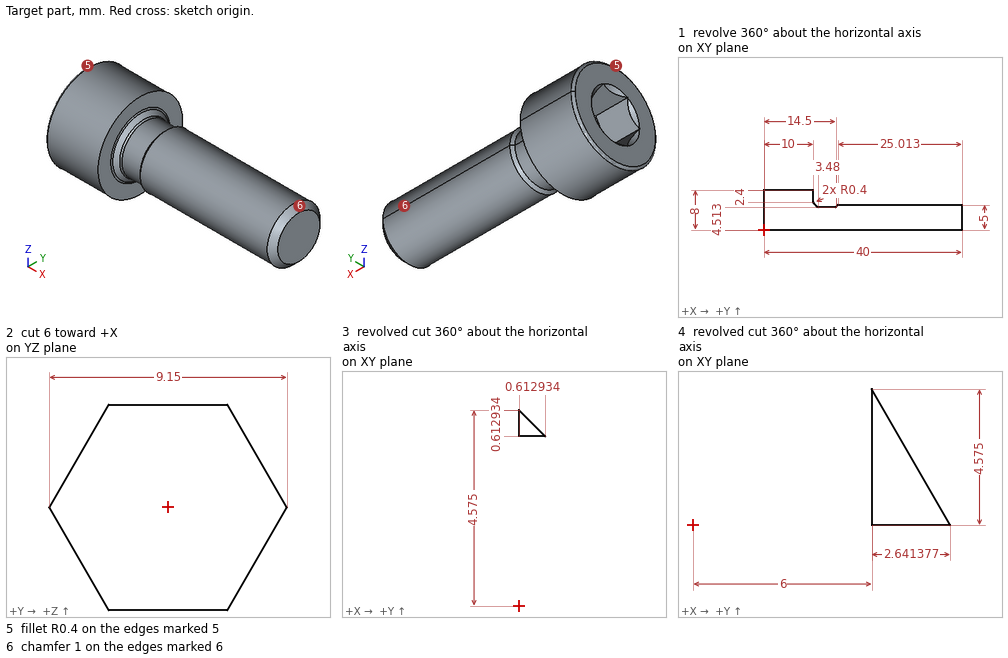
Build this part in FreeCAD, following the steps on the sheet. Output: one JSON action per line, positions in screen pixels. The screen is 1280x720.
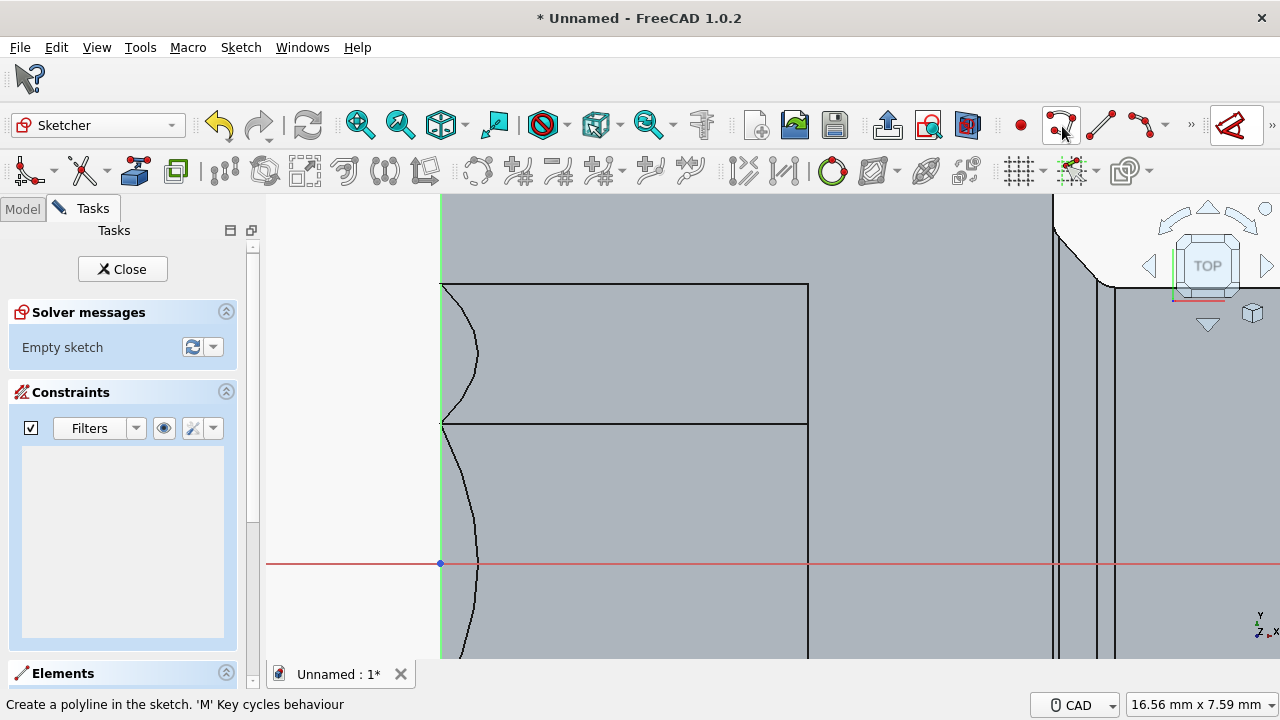
{"action": "left_click", "coordinate": [808, 564]}
{"action": "left_click", "coordinate": [970, 555]}
{"action": "left_click", "coordinate": [808, 284]}
{"action": "left_click", "coordinate": [808, 564]}
{"action": "key", "text": "Escape"}
{"action": "key", "text": "Escape"}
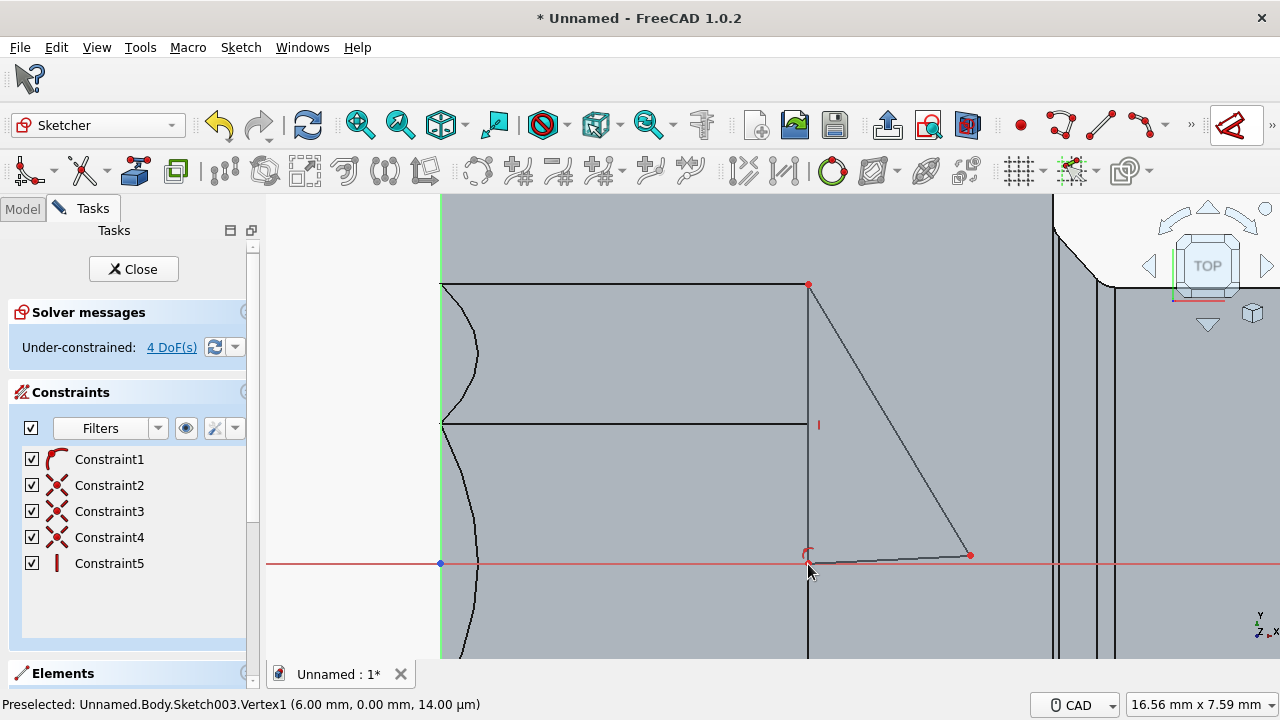
{"action": "left_click", "coordinate": [857, 561]}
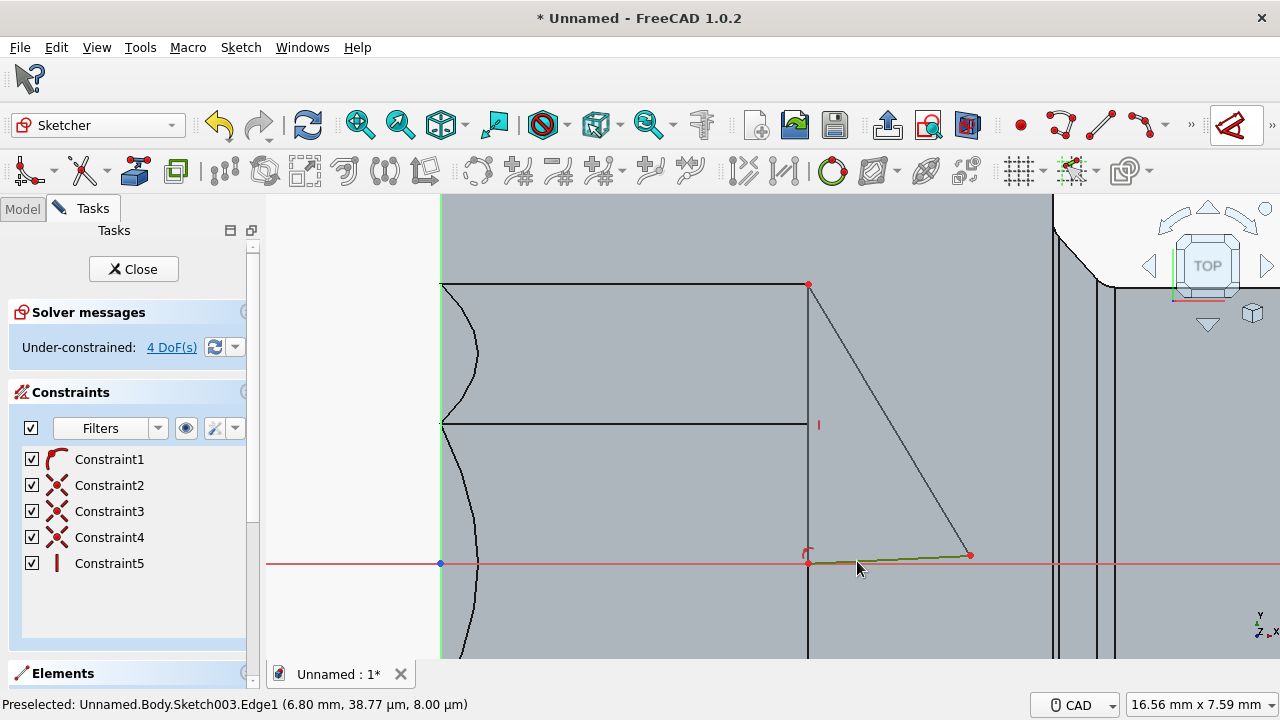
{"action": "key", "text": "h"}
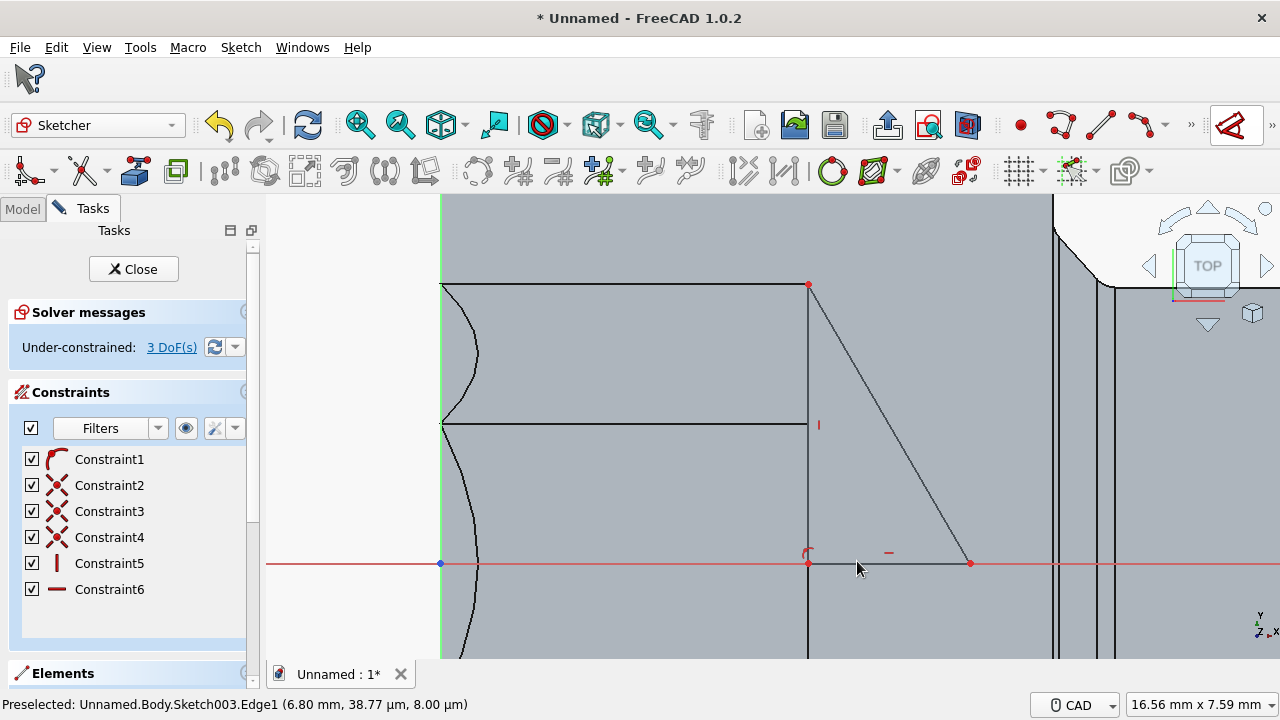
{"action": "left_click", "coordinate": [808, 564]}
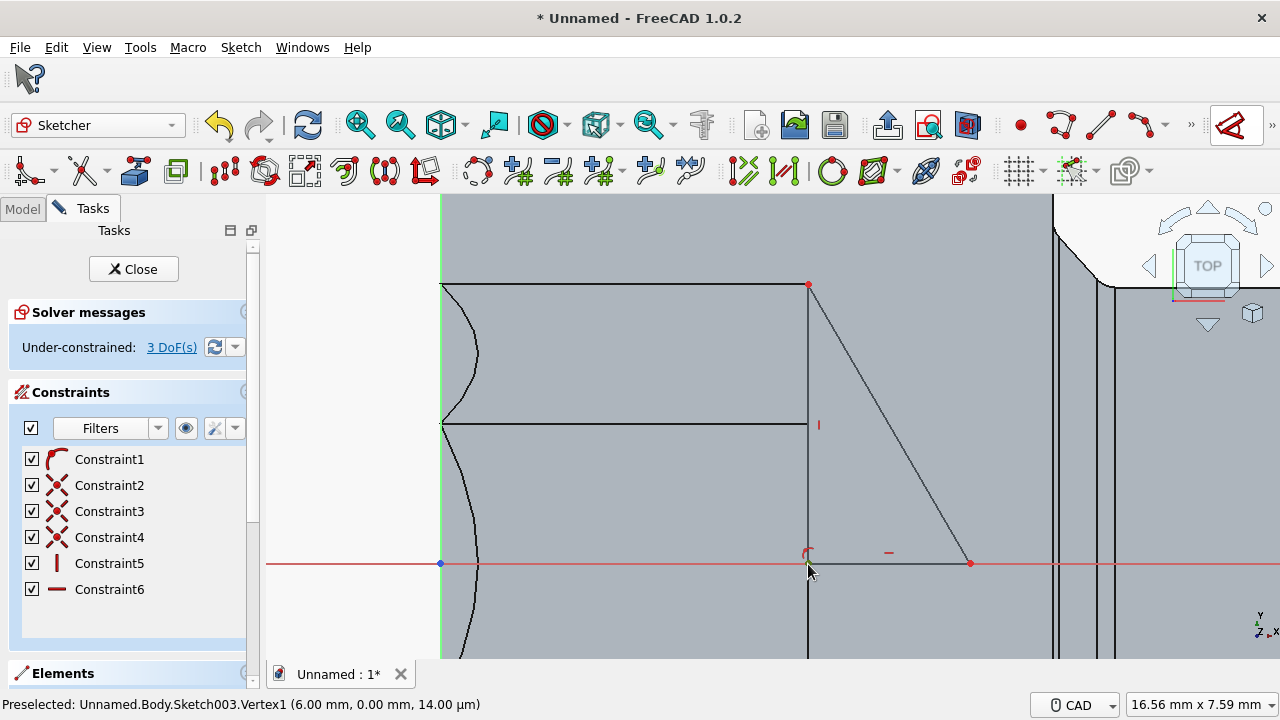
{"action": "left_click", "coordinate": [1258, 126]}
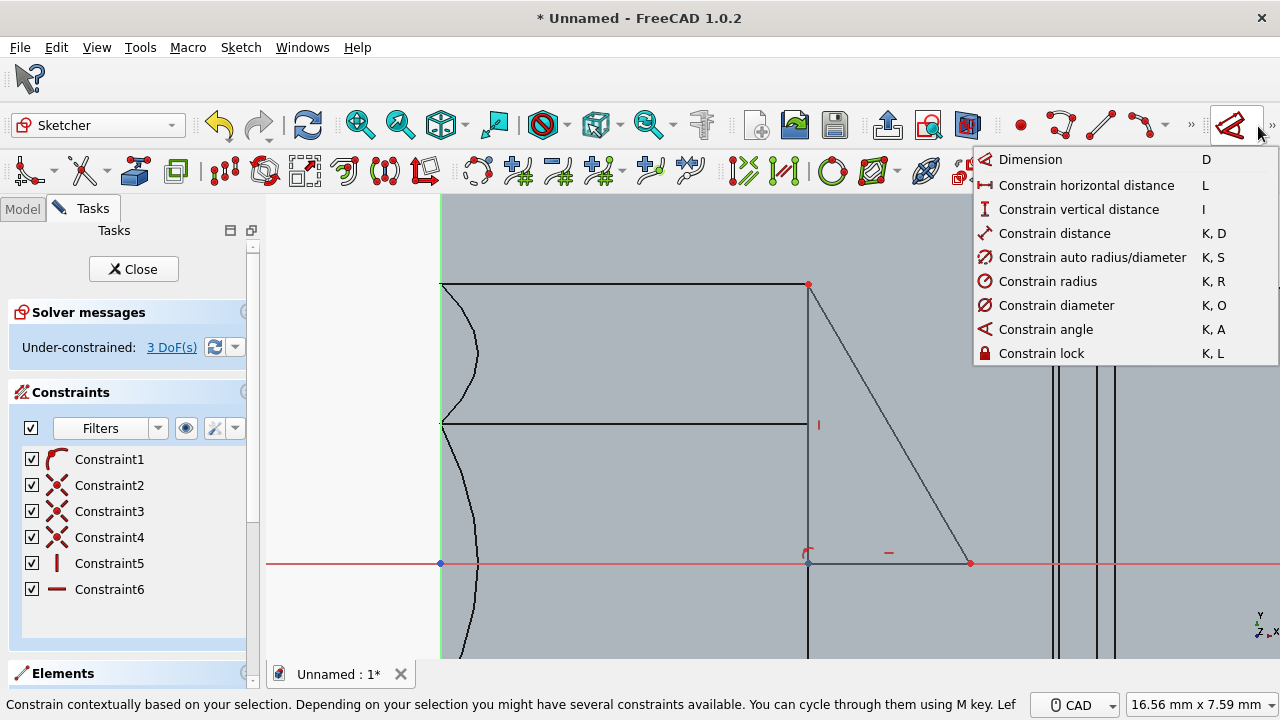
{"action": "left_click", "coordinate": [1126, 185]}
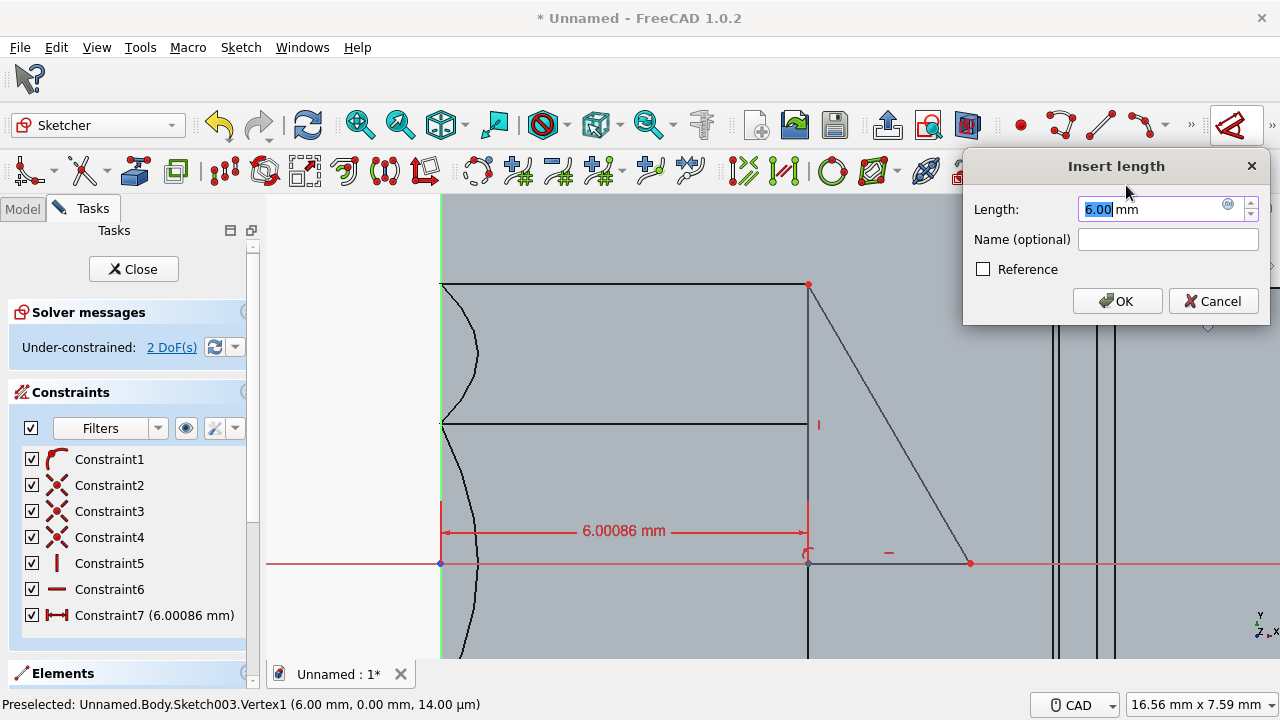
{"action": "type", "text": "6"}
{"action": "key", "text": "Return"}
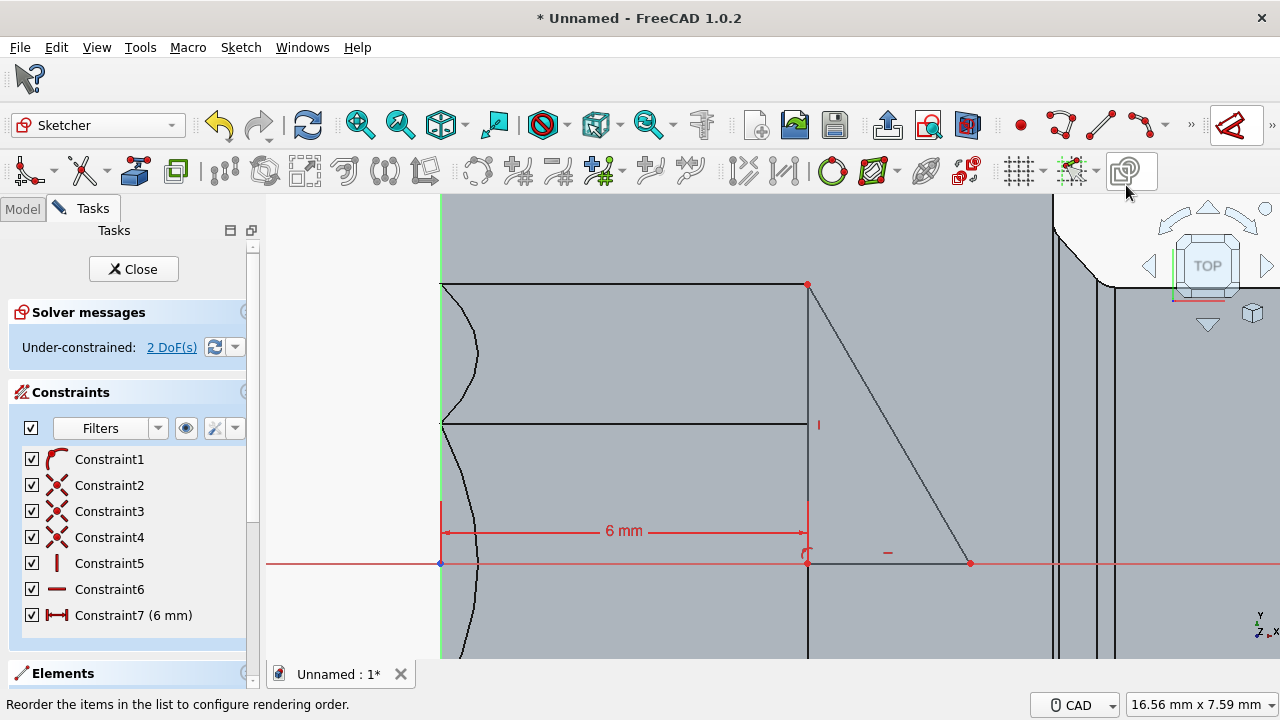
{"action": "left_click", "coordinate": [808, 369]}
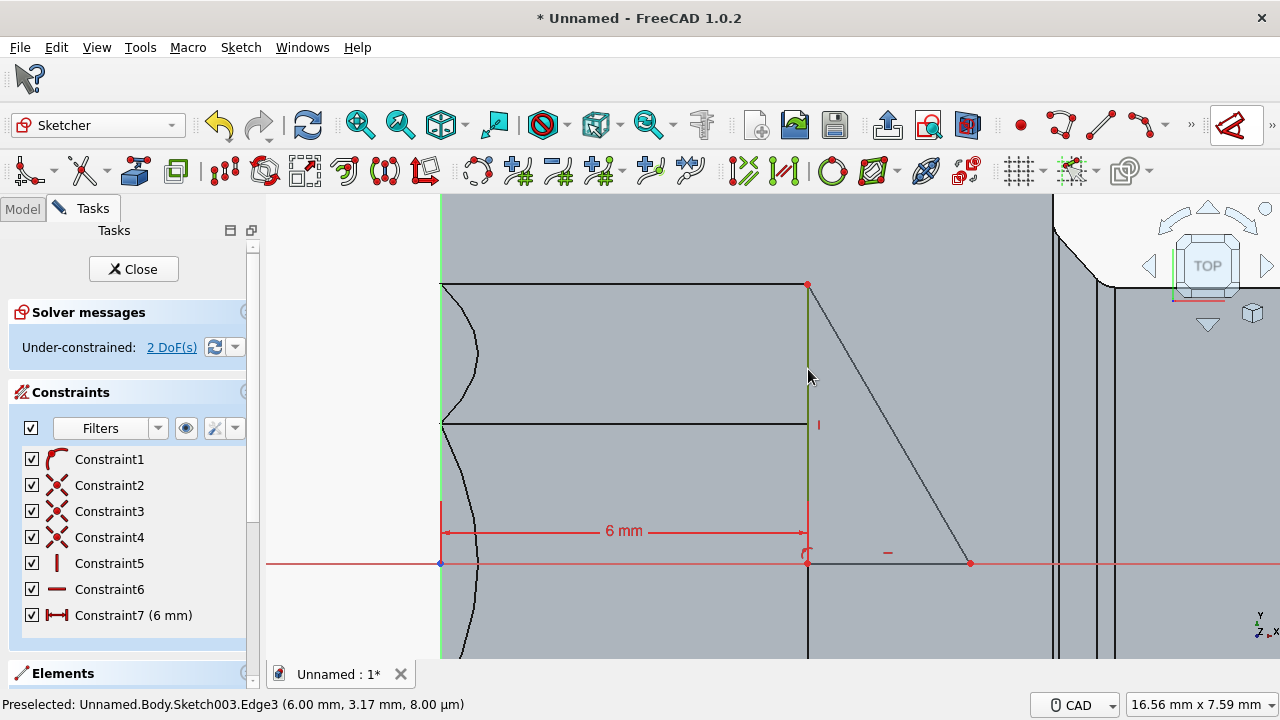
{"action": "left_click", "coordinate": [1258, 126]}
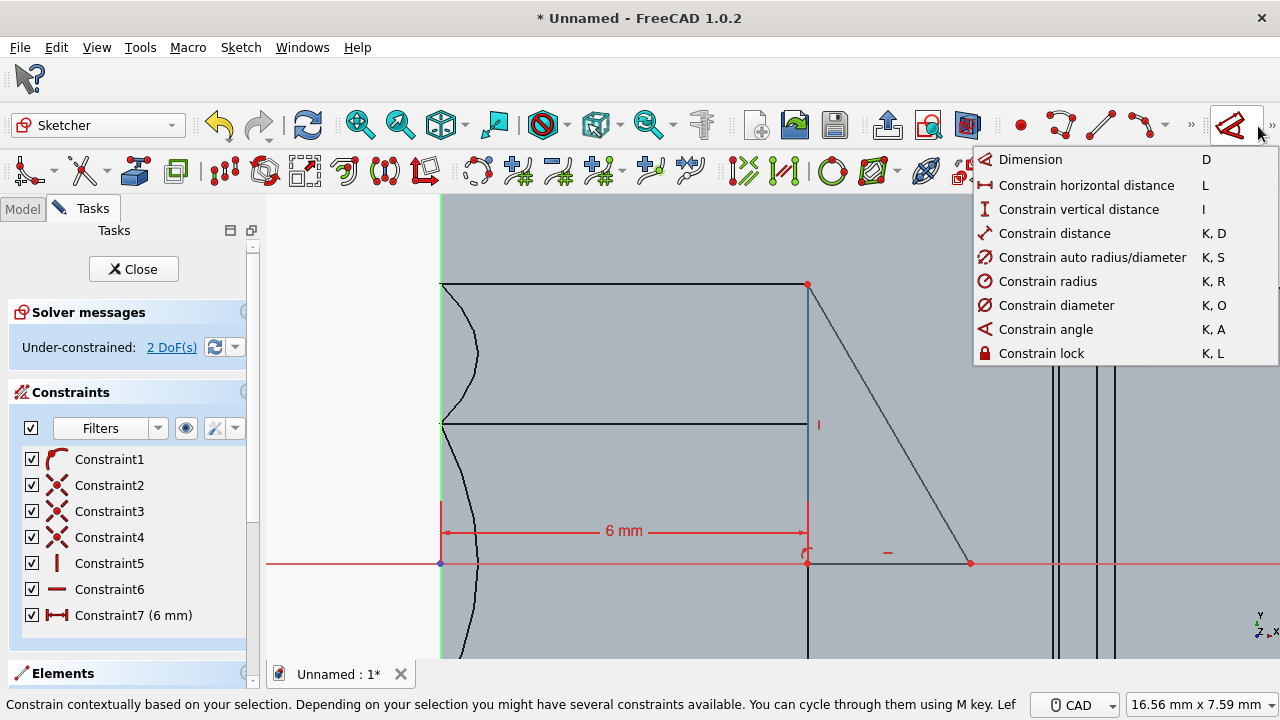
{"action": "left_click", "coordinate": [1126, 209]}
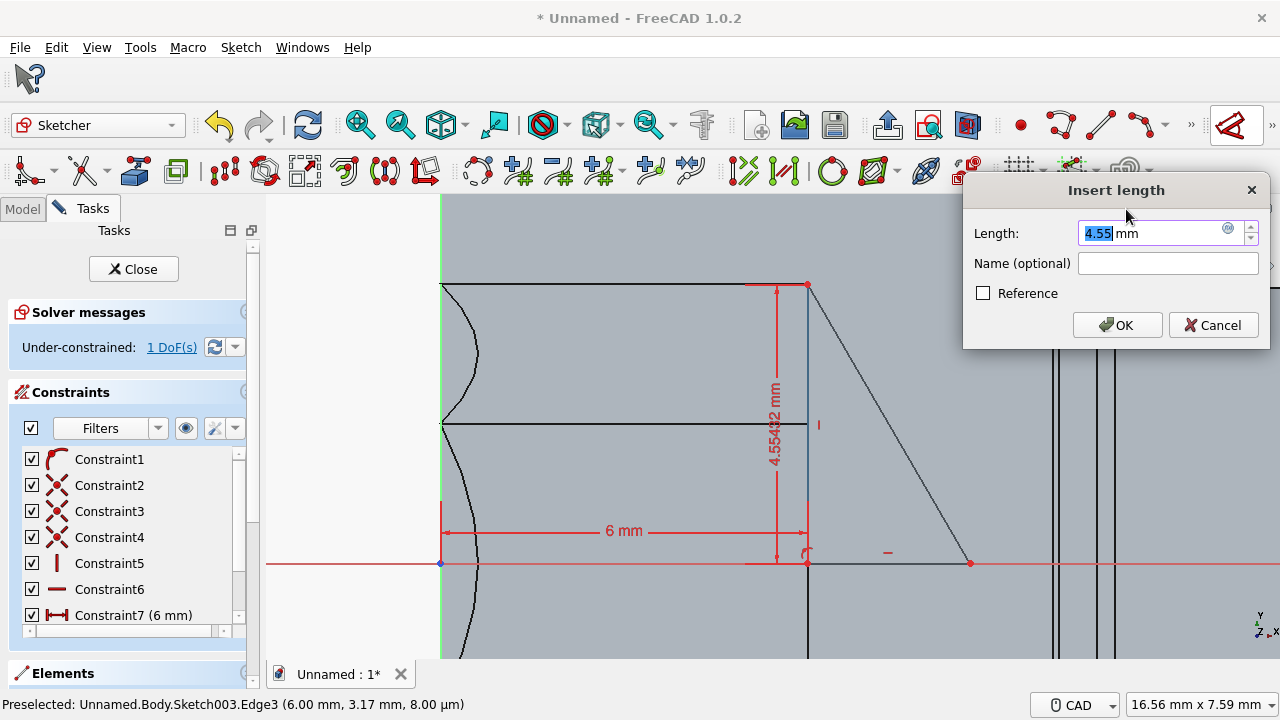
{"action": "type", "text": "4.575"}
{"action": "key", "text": "Return"}